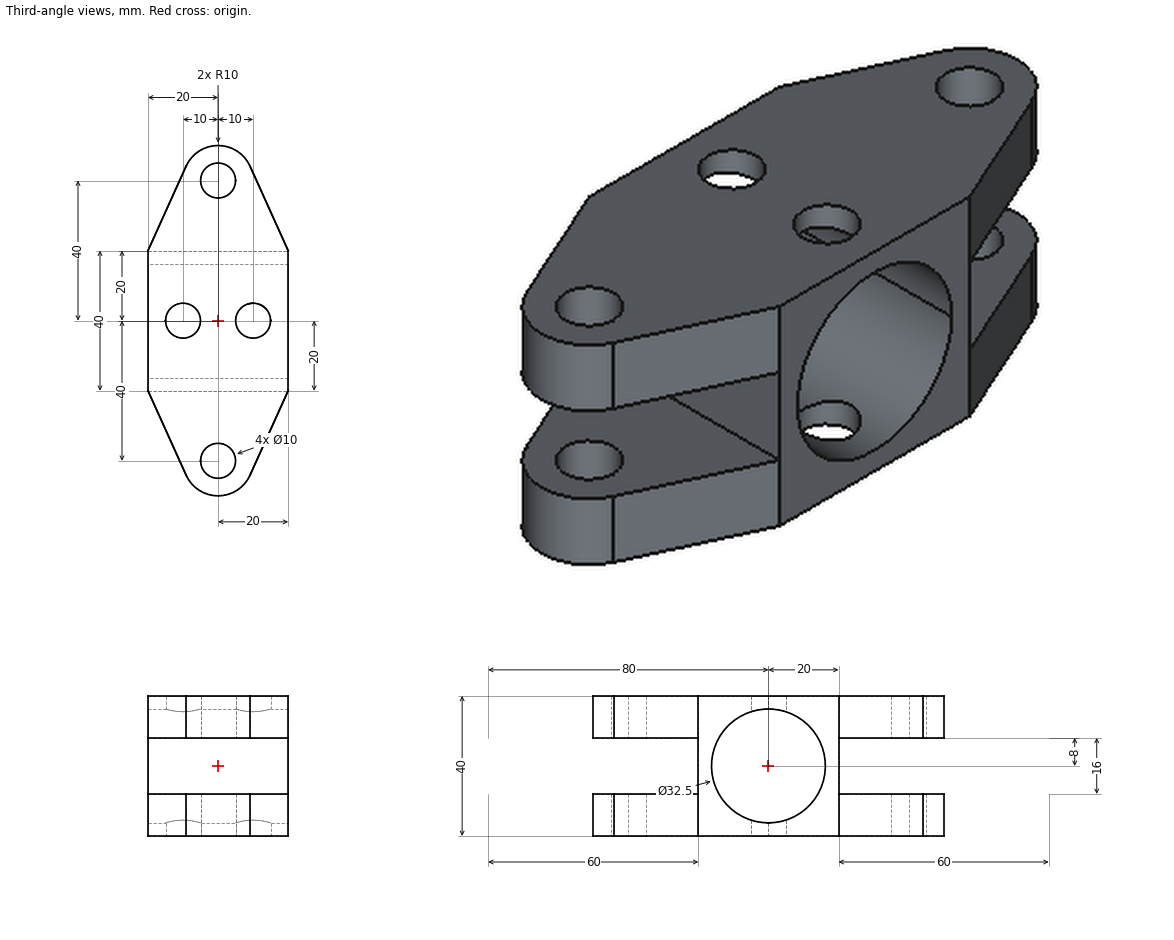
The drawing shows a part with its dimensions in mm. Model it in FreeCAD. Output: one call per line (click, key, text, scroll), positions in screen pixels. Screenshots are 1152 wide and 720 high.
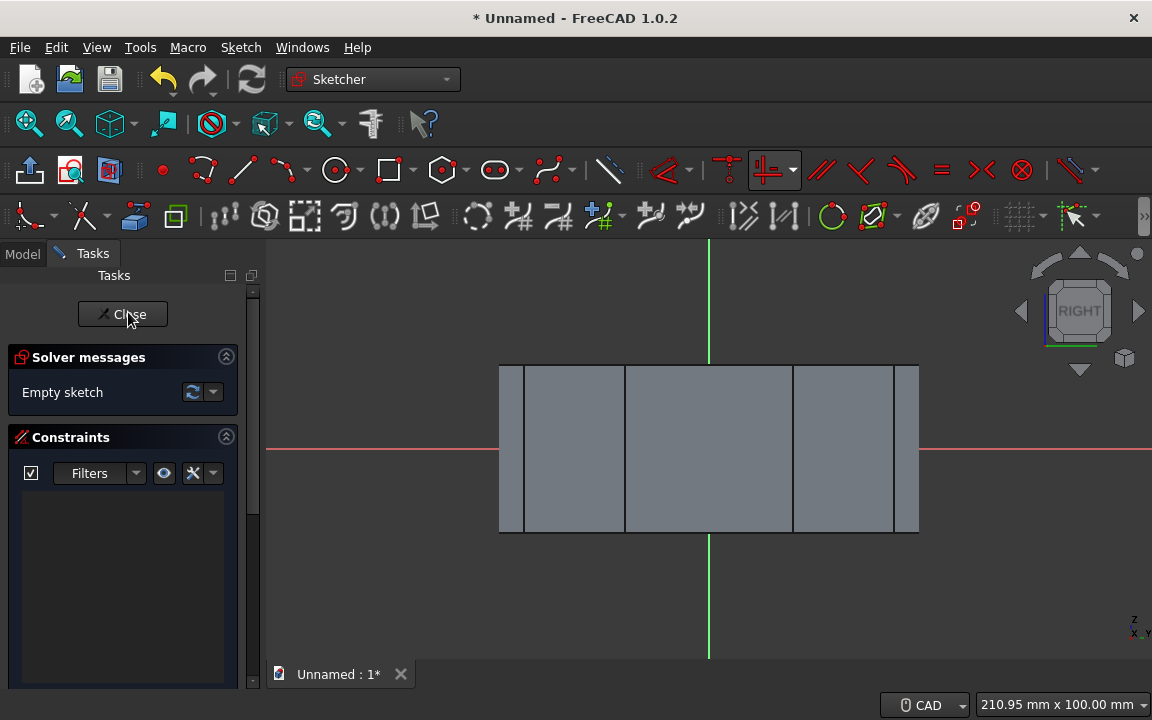
click(110, 170)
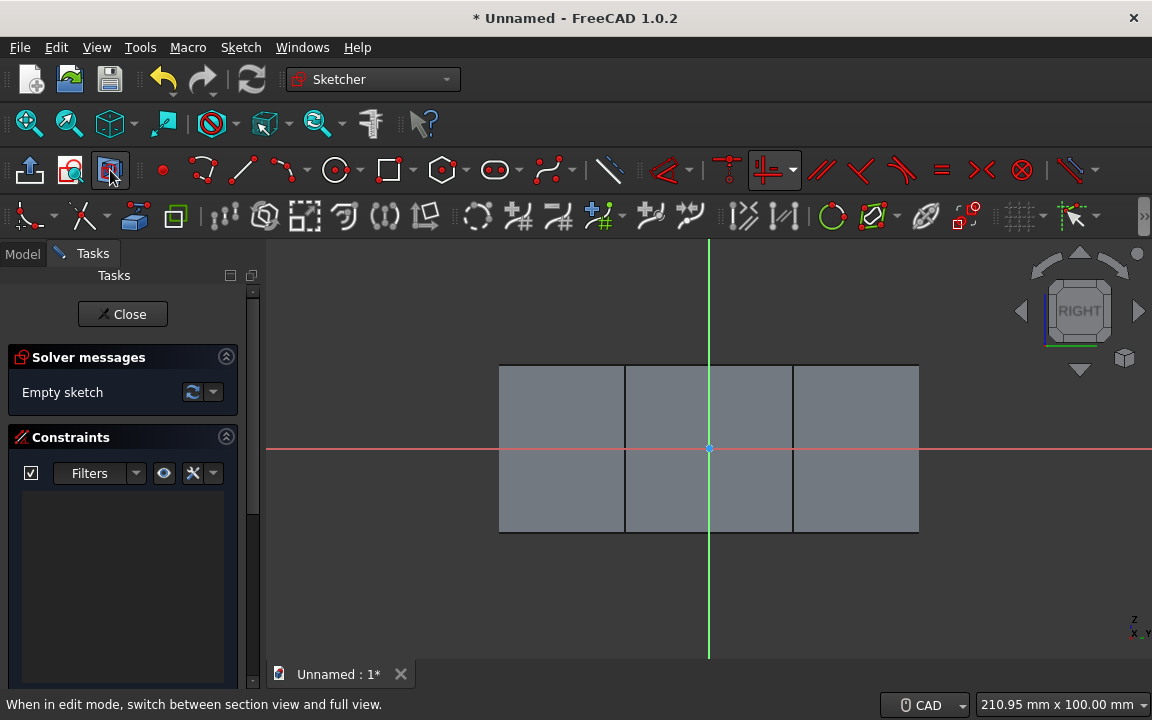
scroll(501, 449, down, 2)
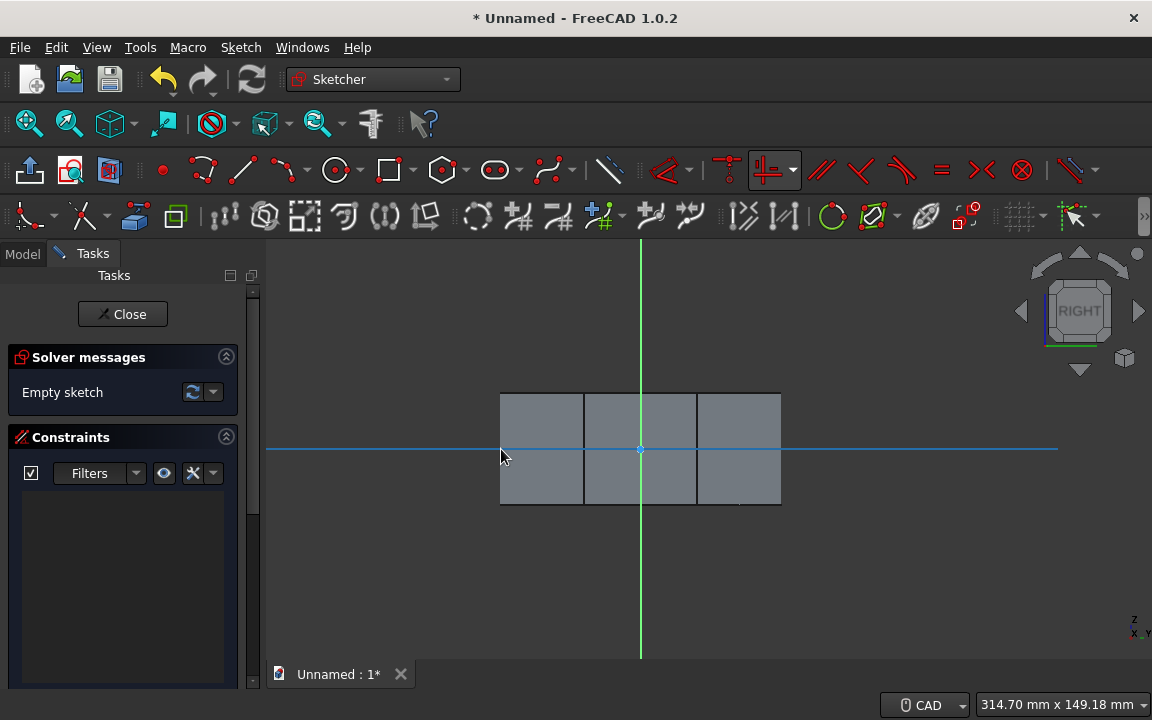
click(390, 170)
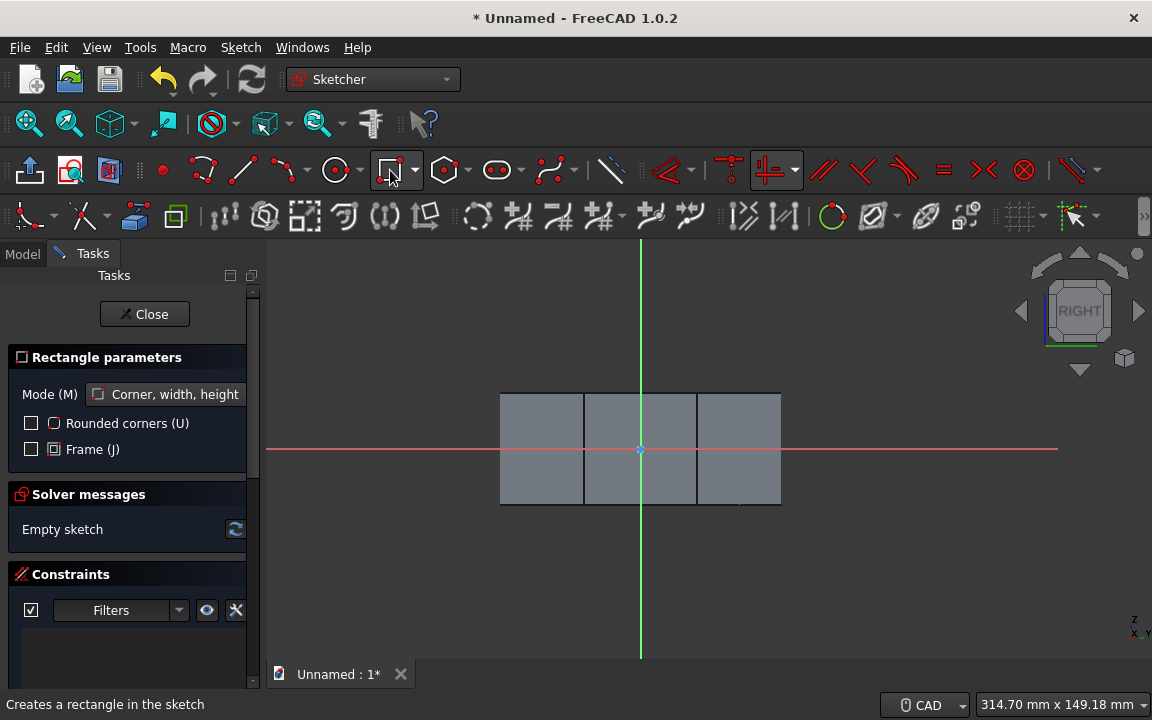
click(697, 427)
move(866, 472)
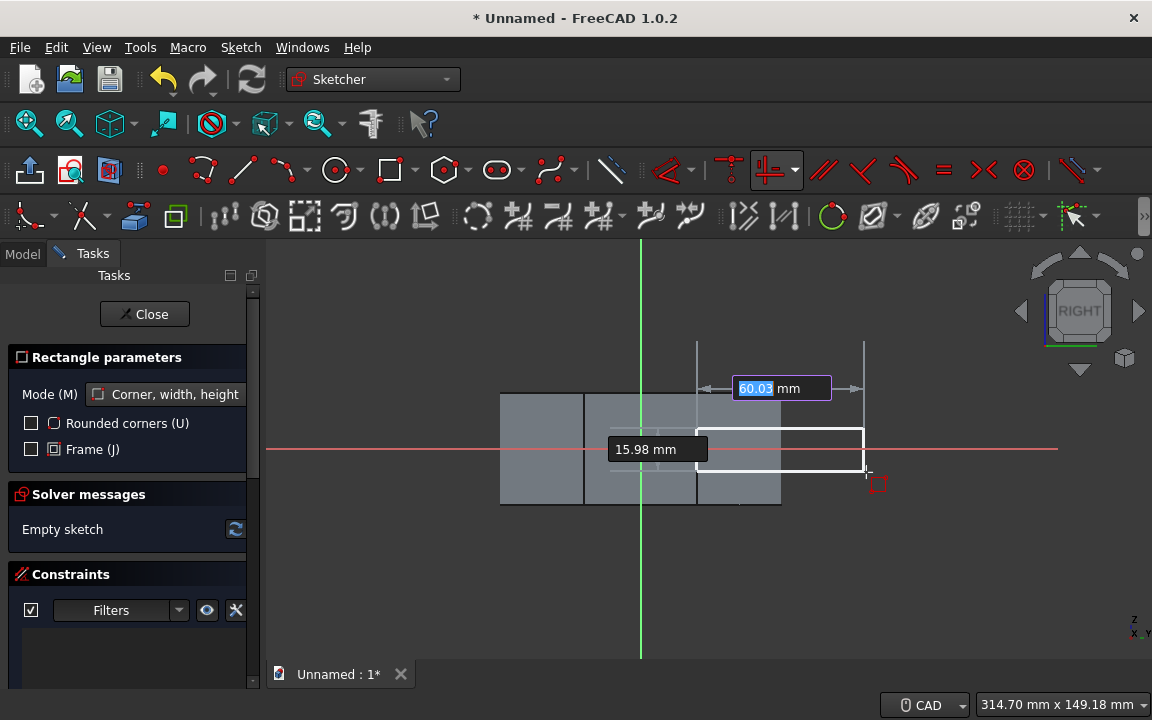
text(60)
key(Tab)
text(16)
key(Return)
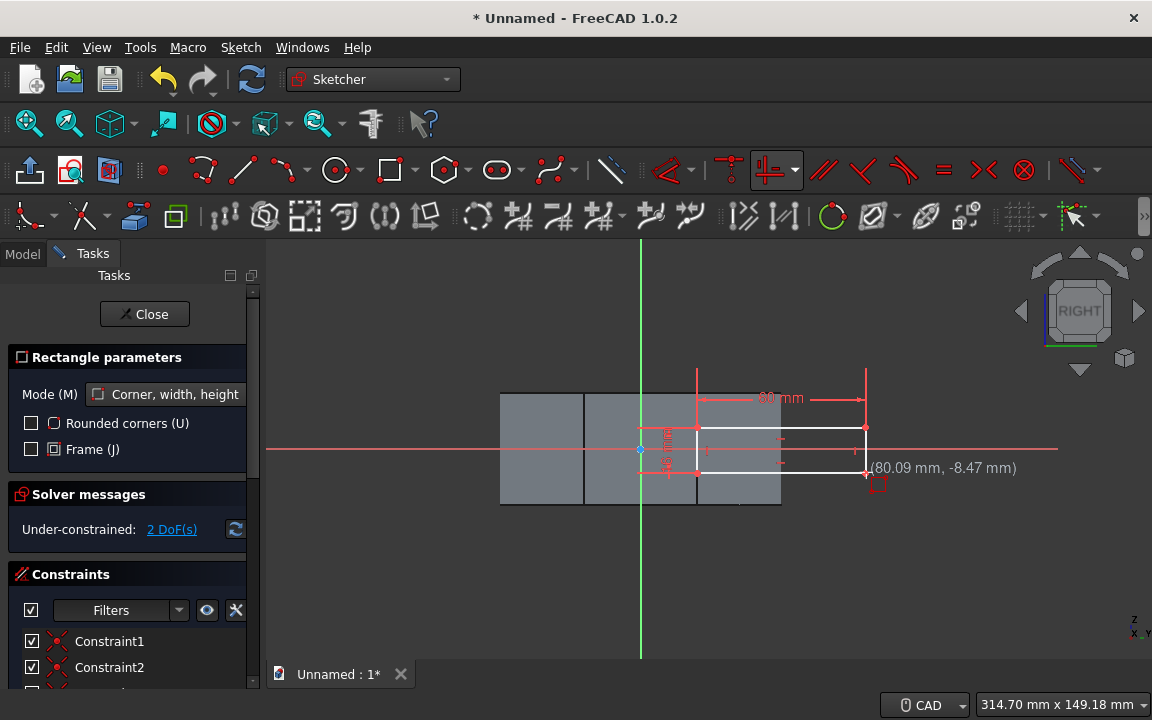
click(415, 427)
move(584, 472)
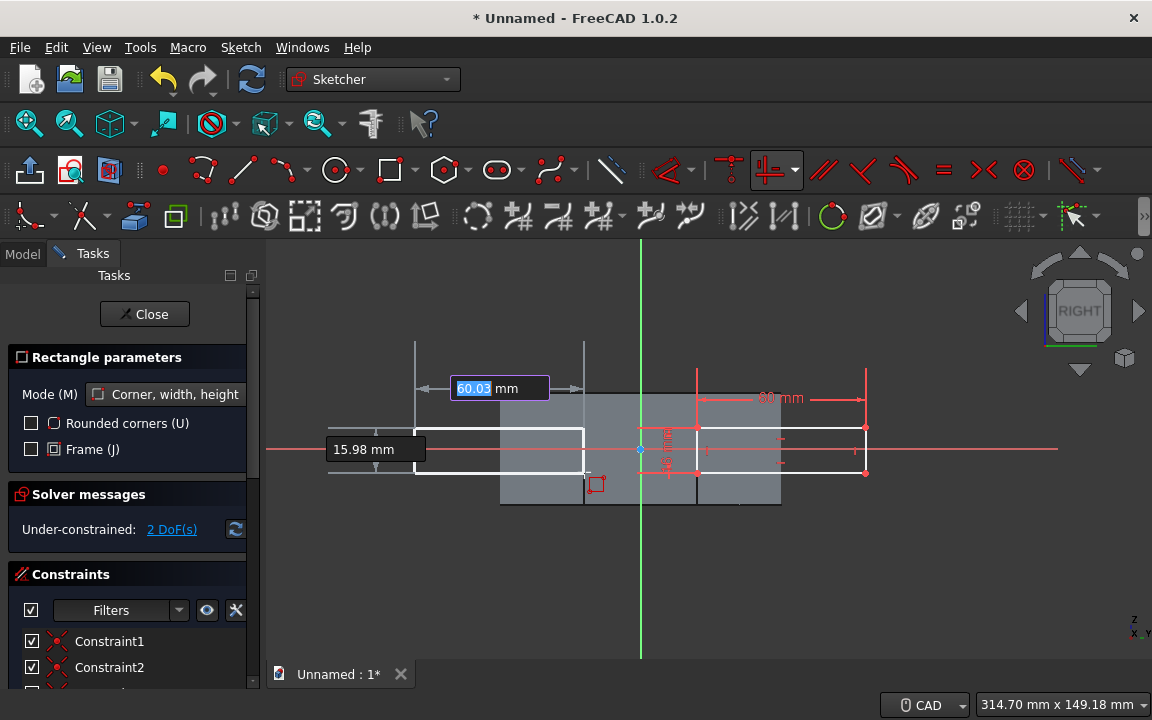
text(60)
key(Tab)
text(16)
key(Return)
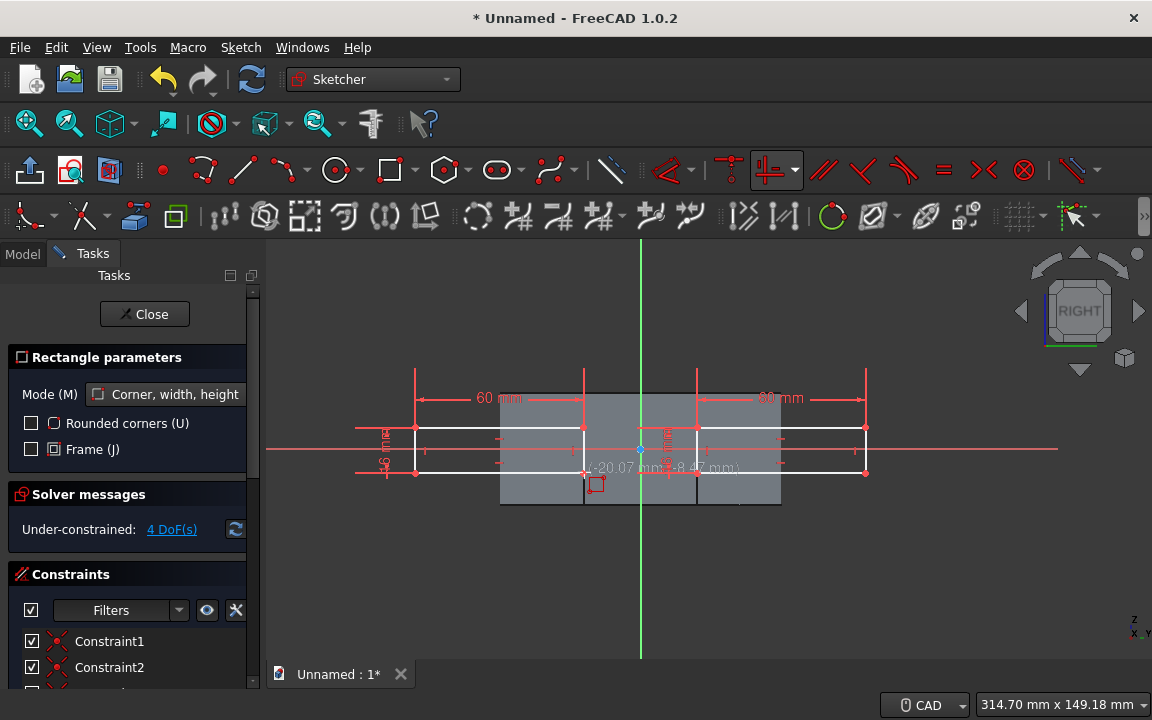
click(336, 170)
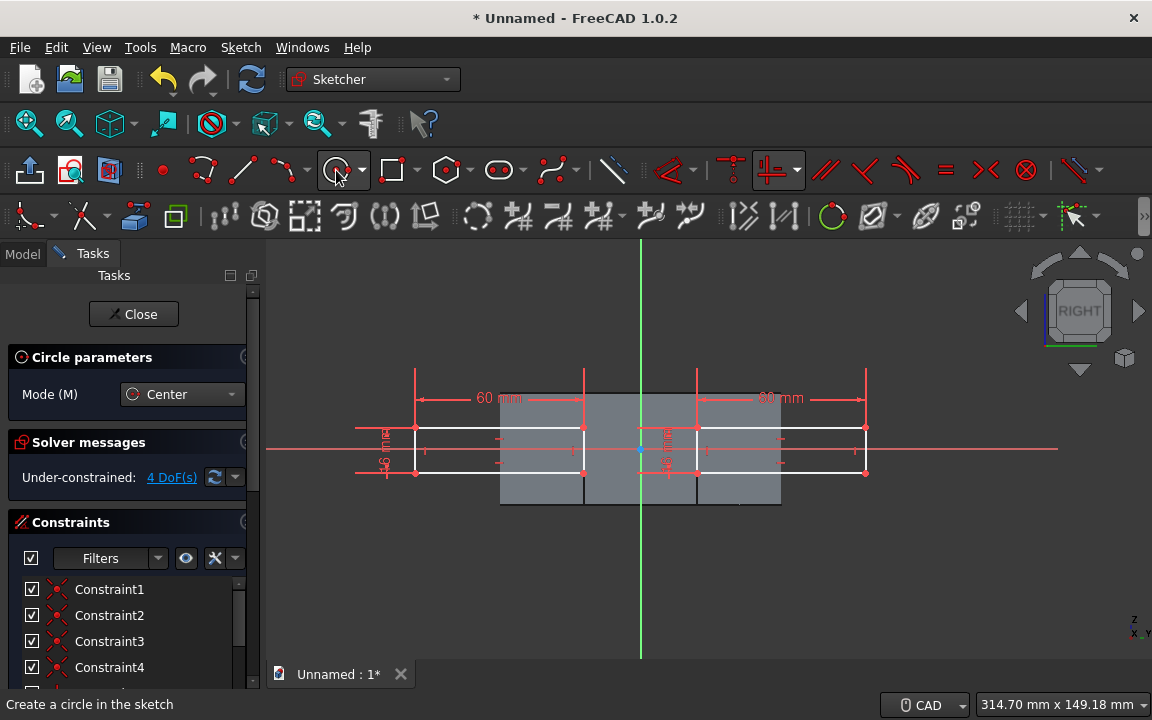
click(641, 449)
move(673, 417)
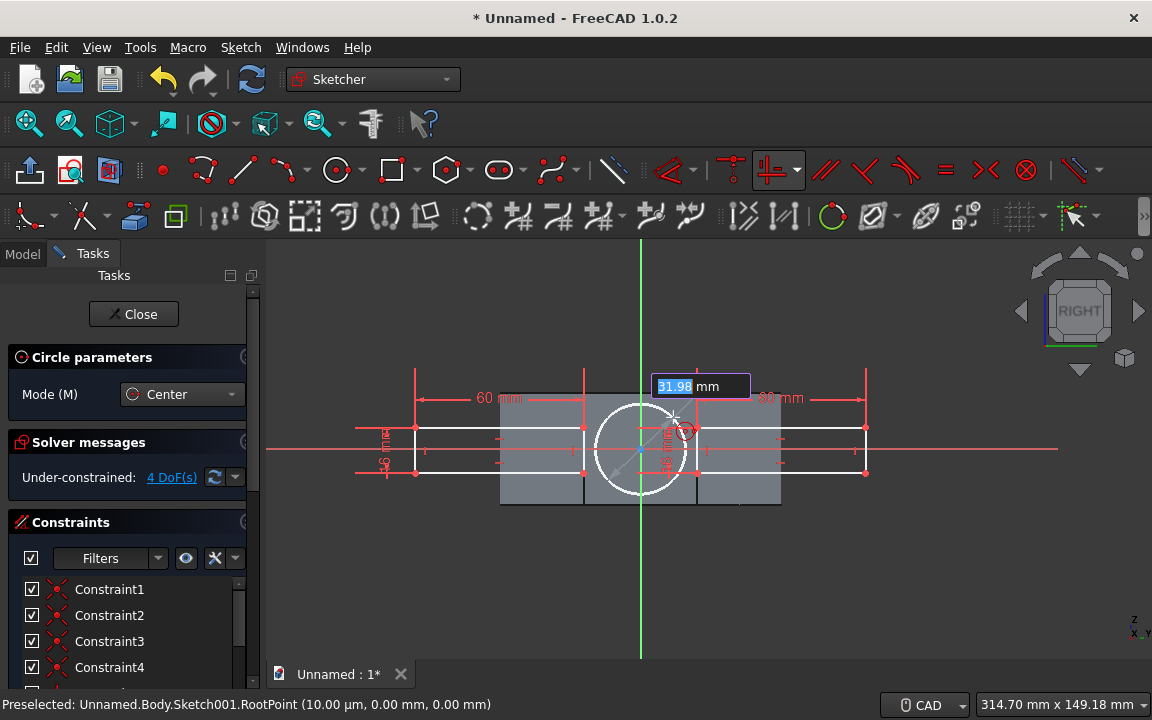
text(32.5)
key(Return)
key(Escape)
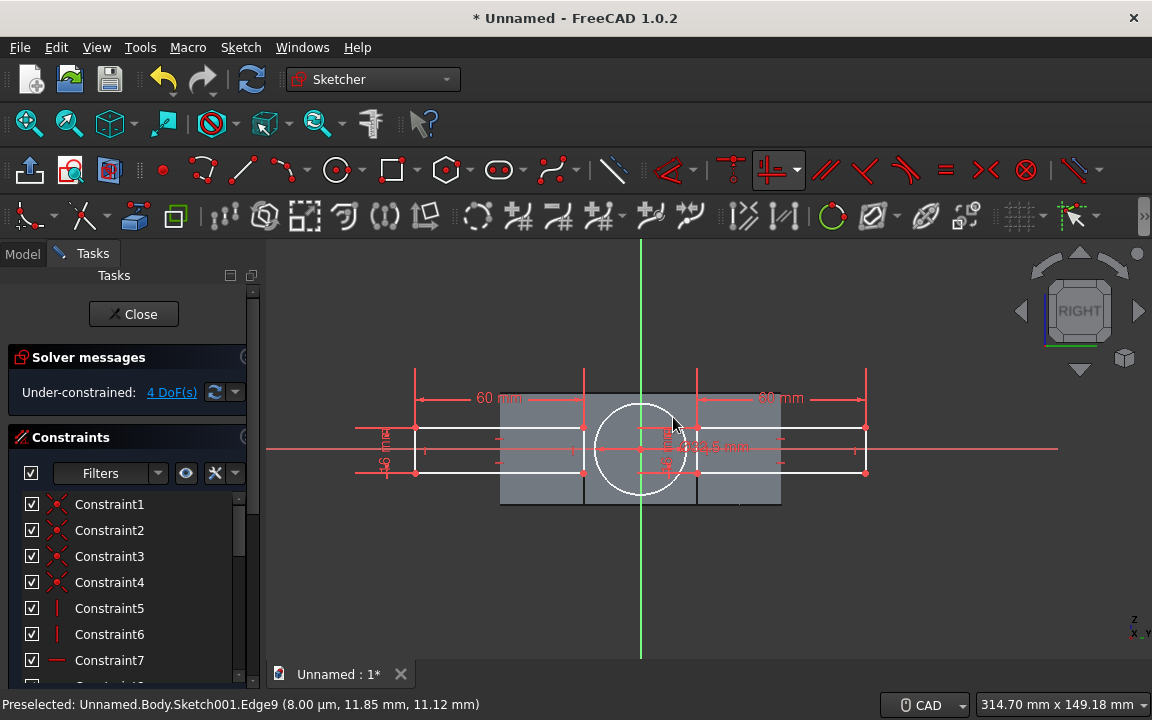
click(668, 170)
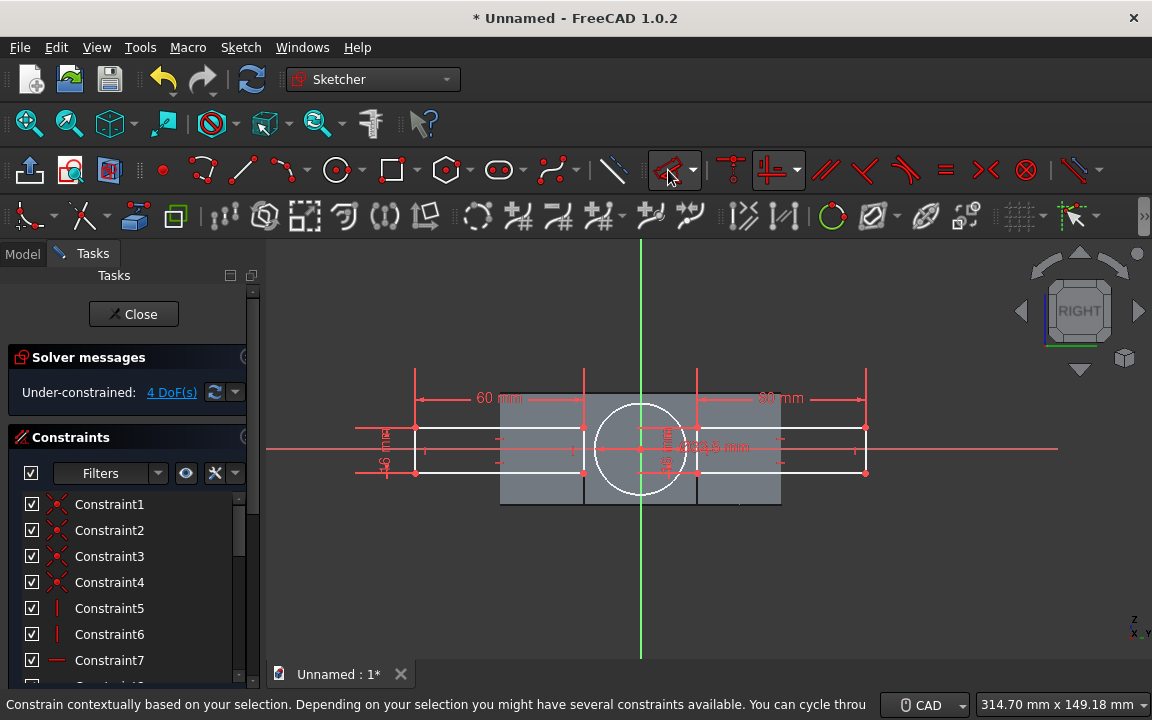
scroll(697, 428, up, 3)